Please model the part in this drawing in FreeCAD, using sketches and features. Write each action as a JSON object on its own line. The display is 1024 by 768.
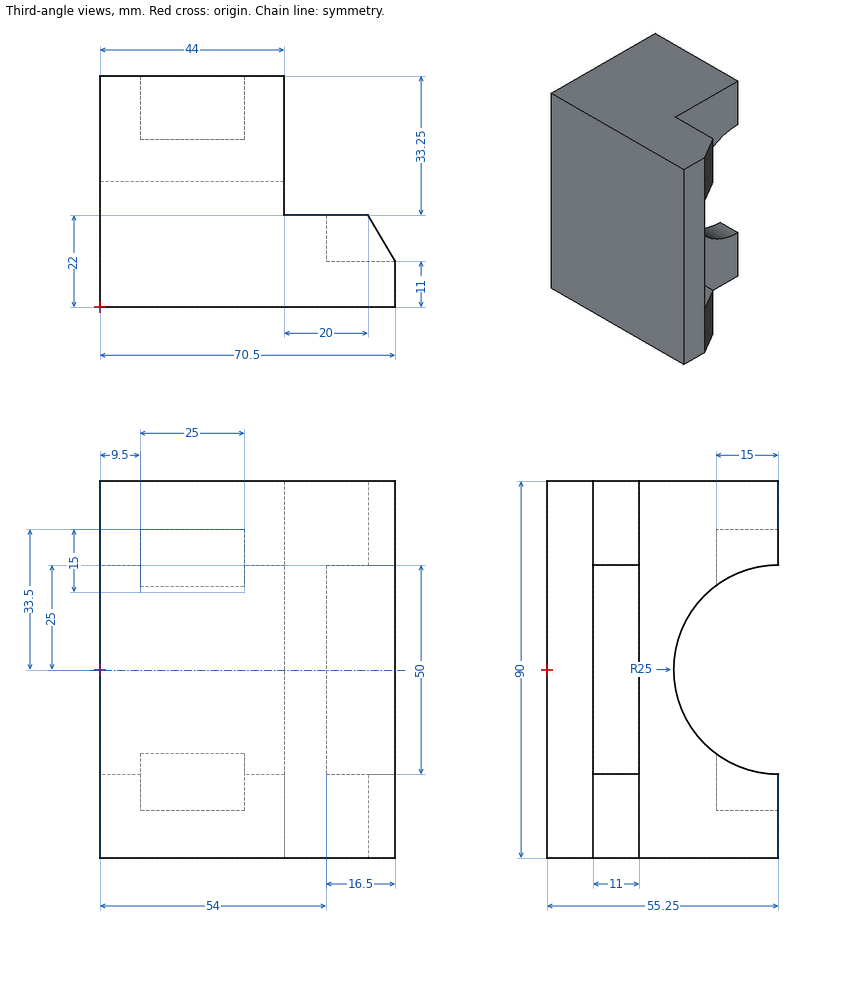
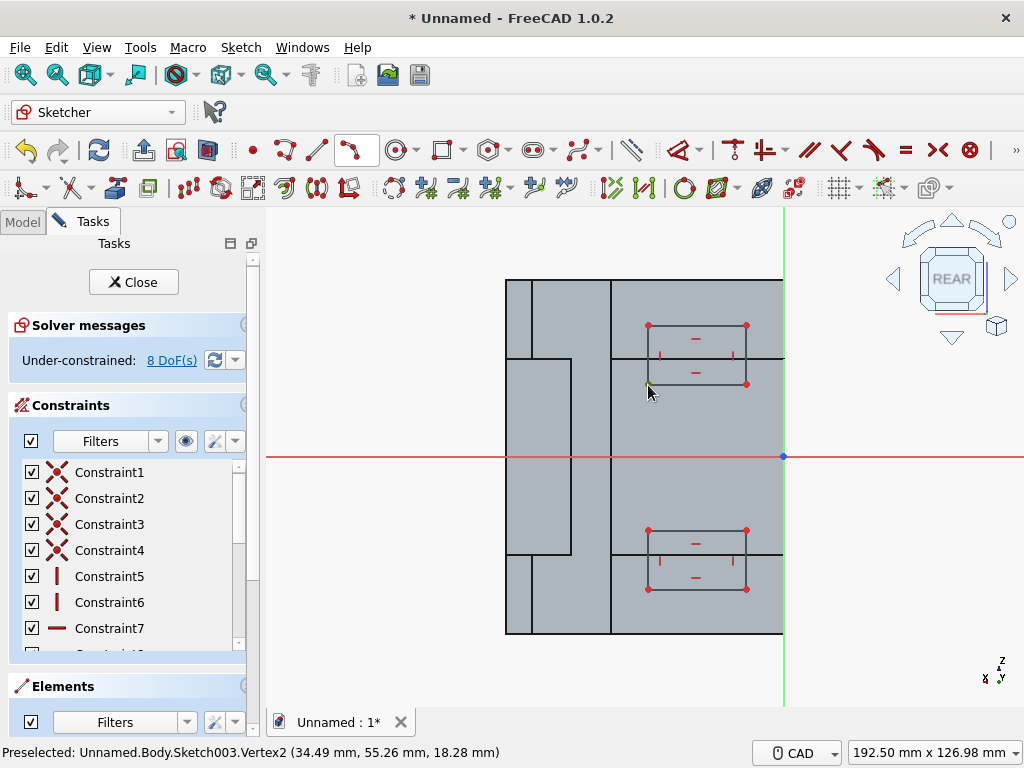
{"action": "left_click", "coordinate": [648, 531]}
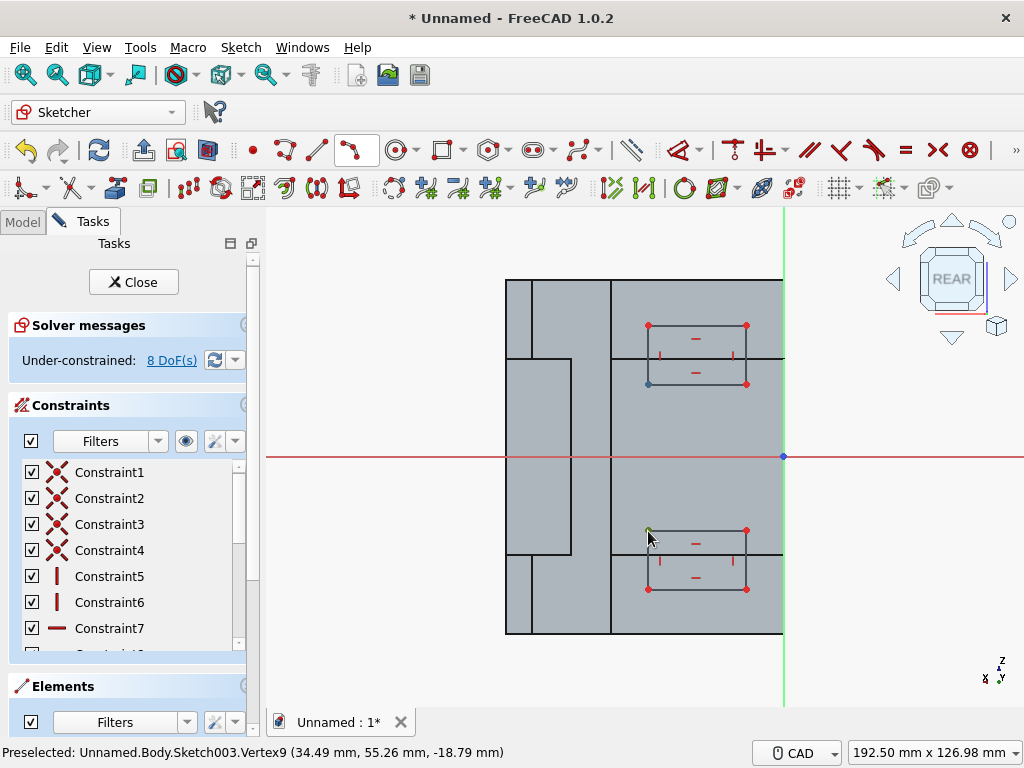
{"action": "left_click", "coordinate": [334, 457]}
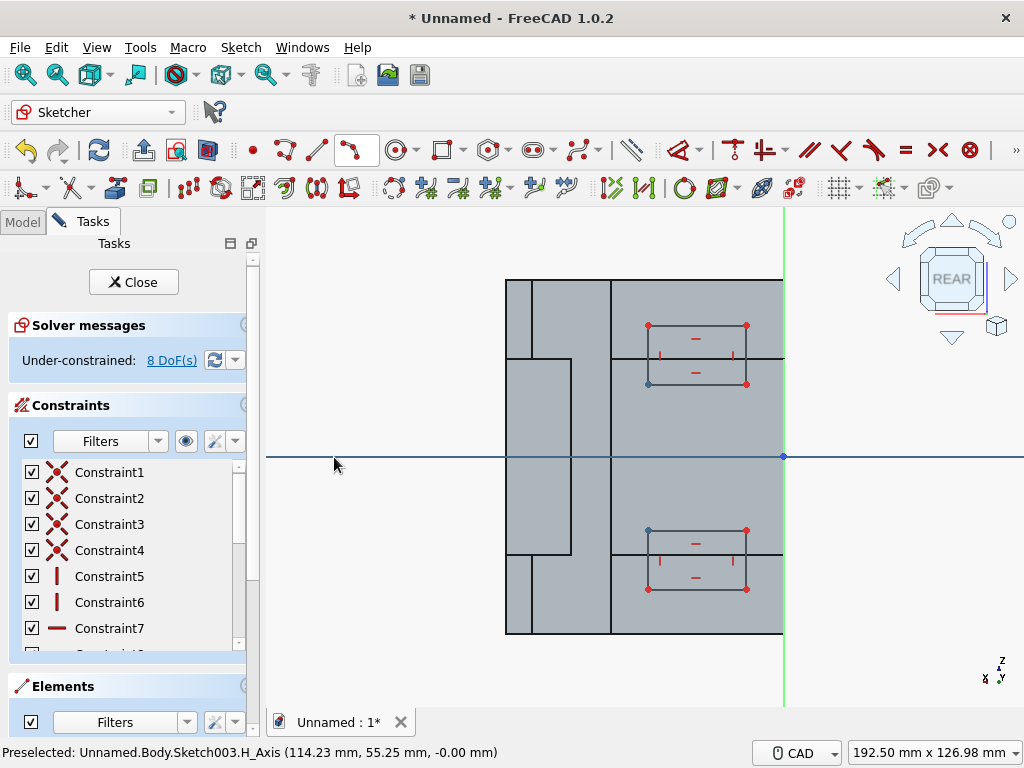
{"action": "left_click", "coordinate": [938, 150]}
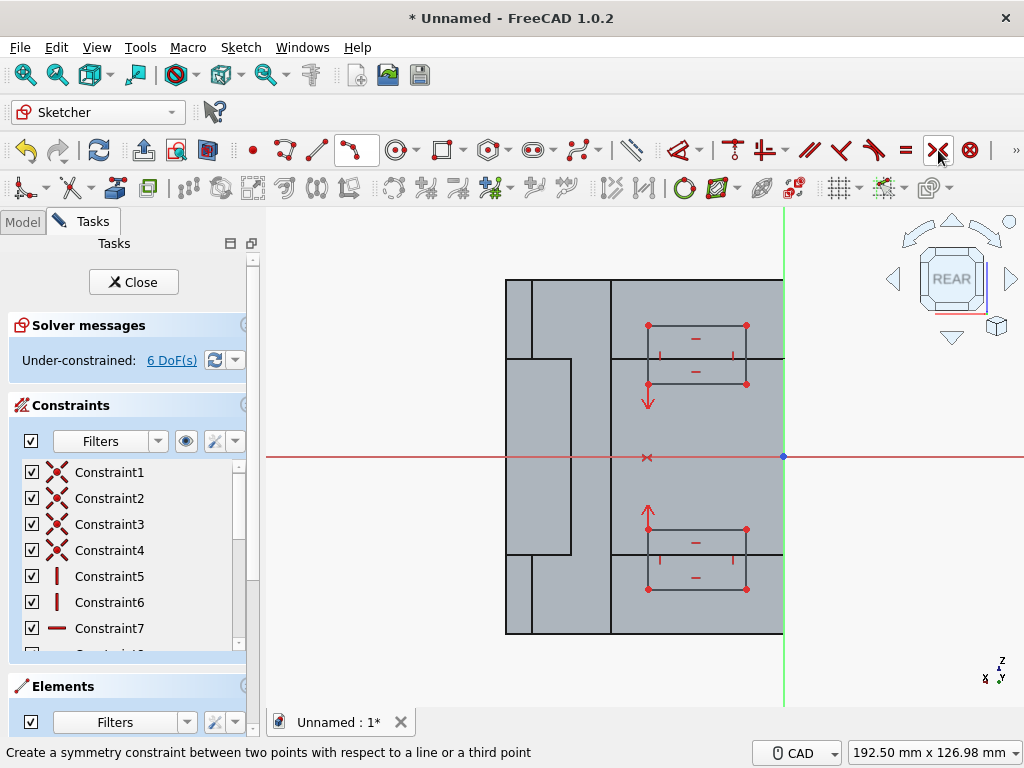
{"action": "left_click", "coordinate": [746, 326]}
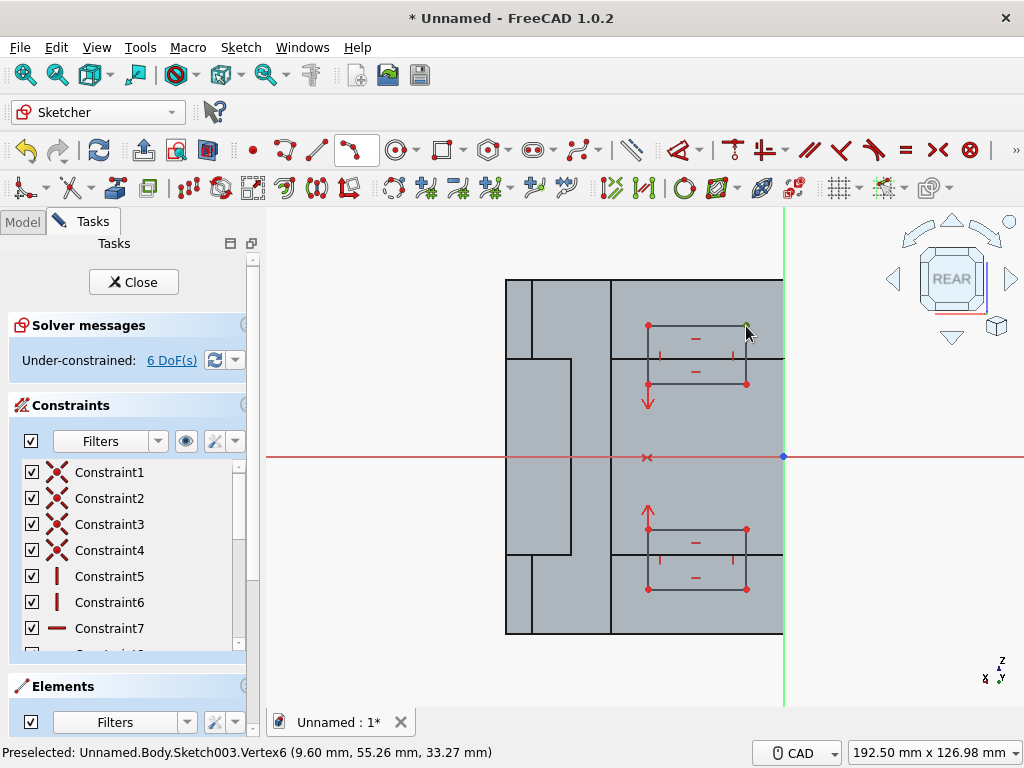
{"action": "left_click", "coordinate": [746, 590]}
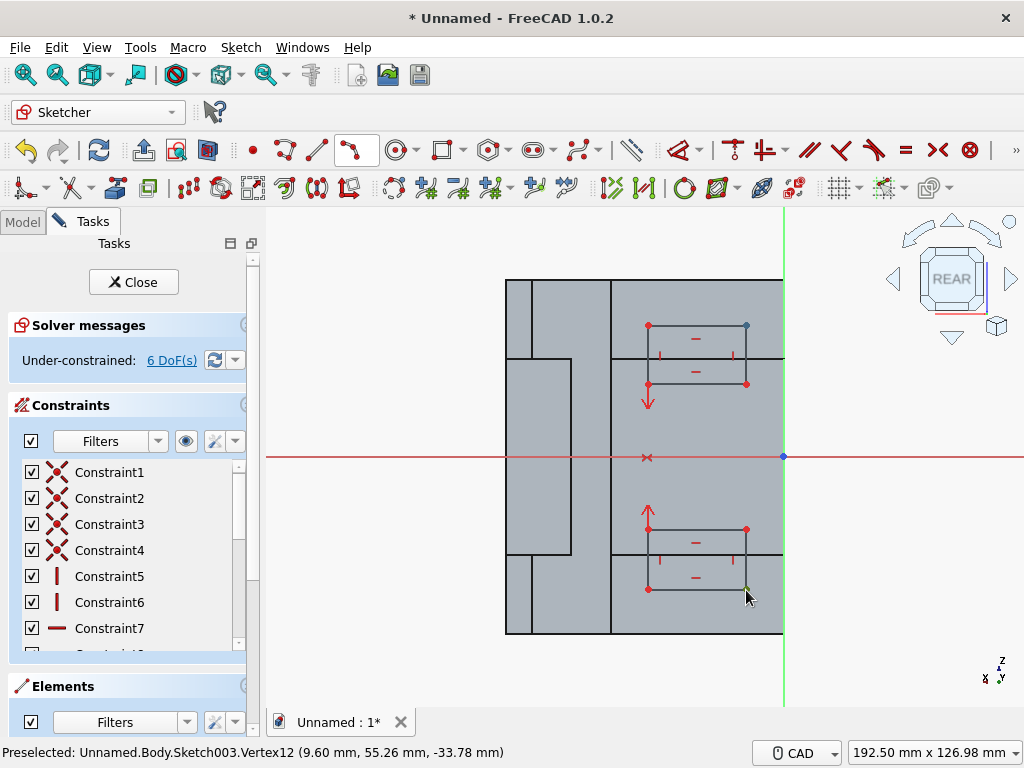
{"action": "left_click", "coordinate": [334, 457]}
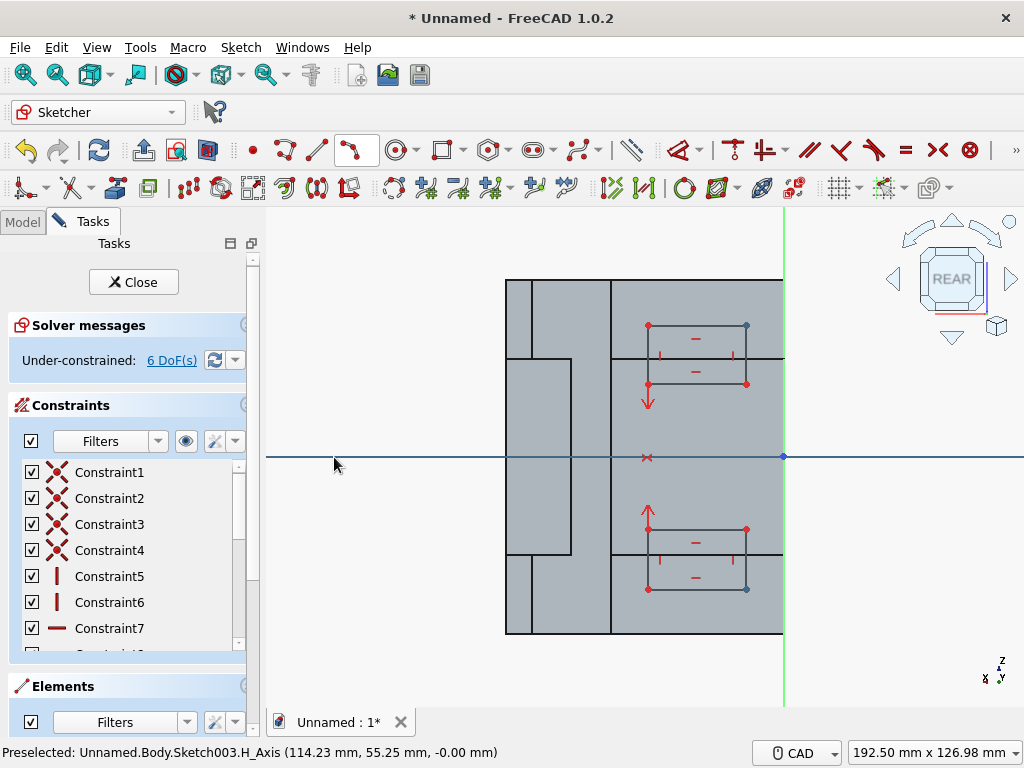
{"action": "left_click", "coordinate": [938, 150]}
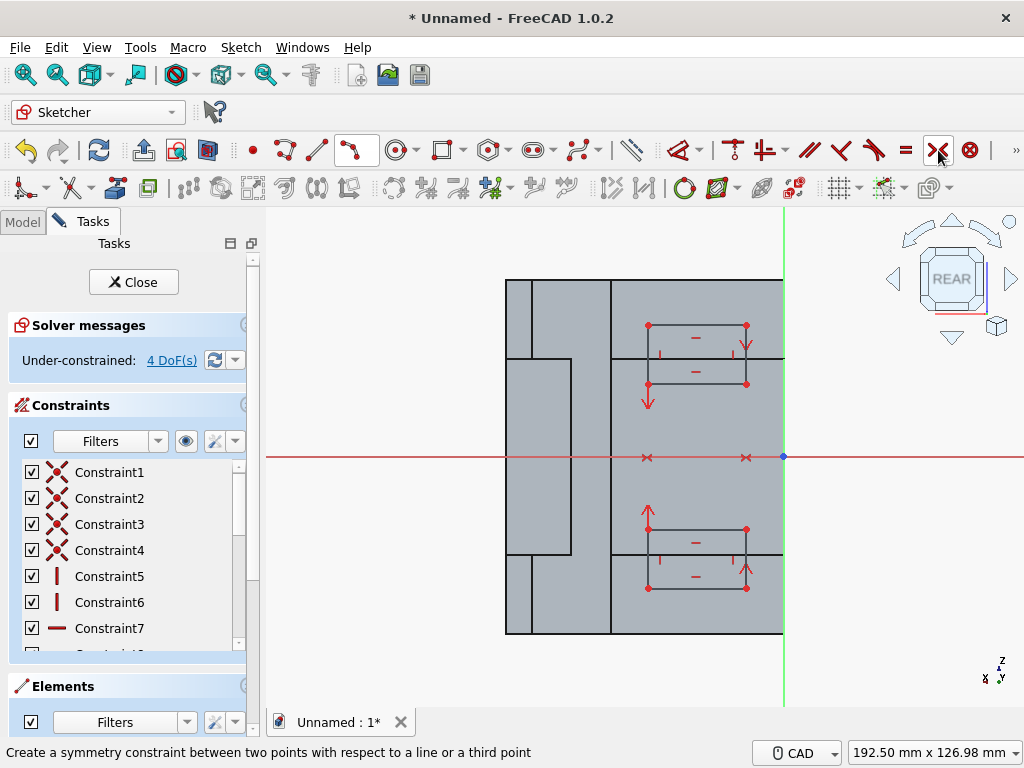
{"action": "left_click", "coordinate": [678, 150]}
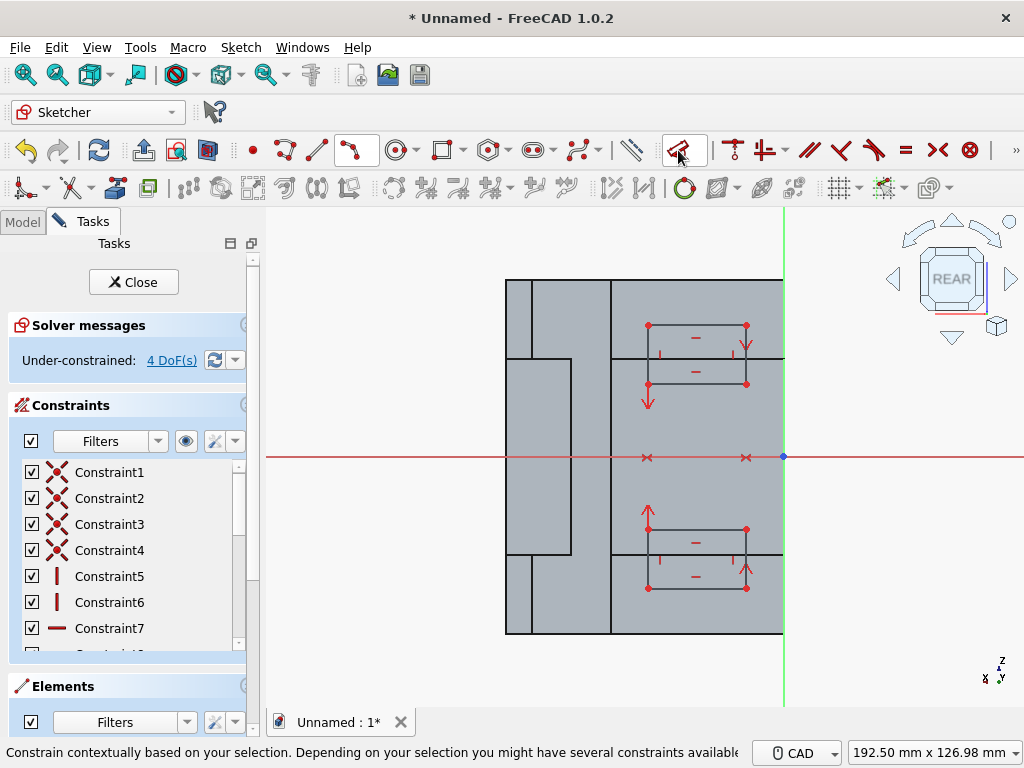
{"action": "left_click", "coordinate": [648, 343]}
{"action": "left_click", "coordinate": [614, 355]}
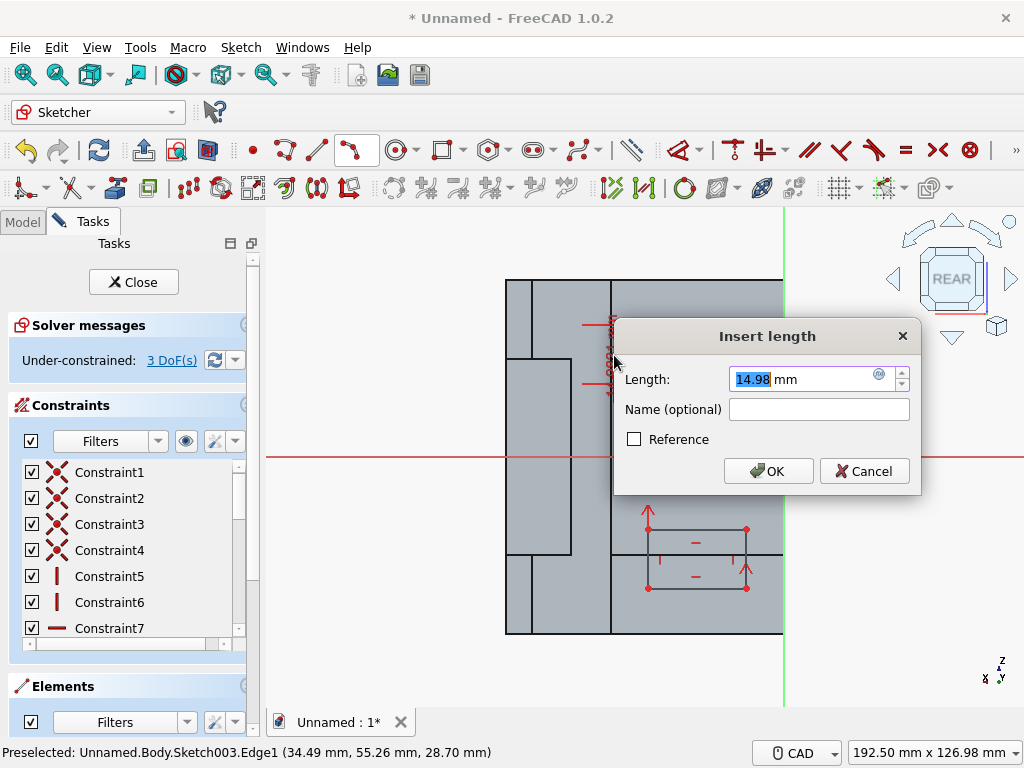
{"action": "type", "text": "15"}
{"action": "key", "text": "Return"}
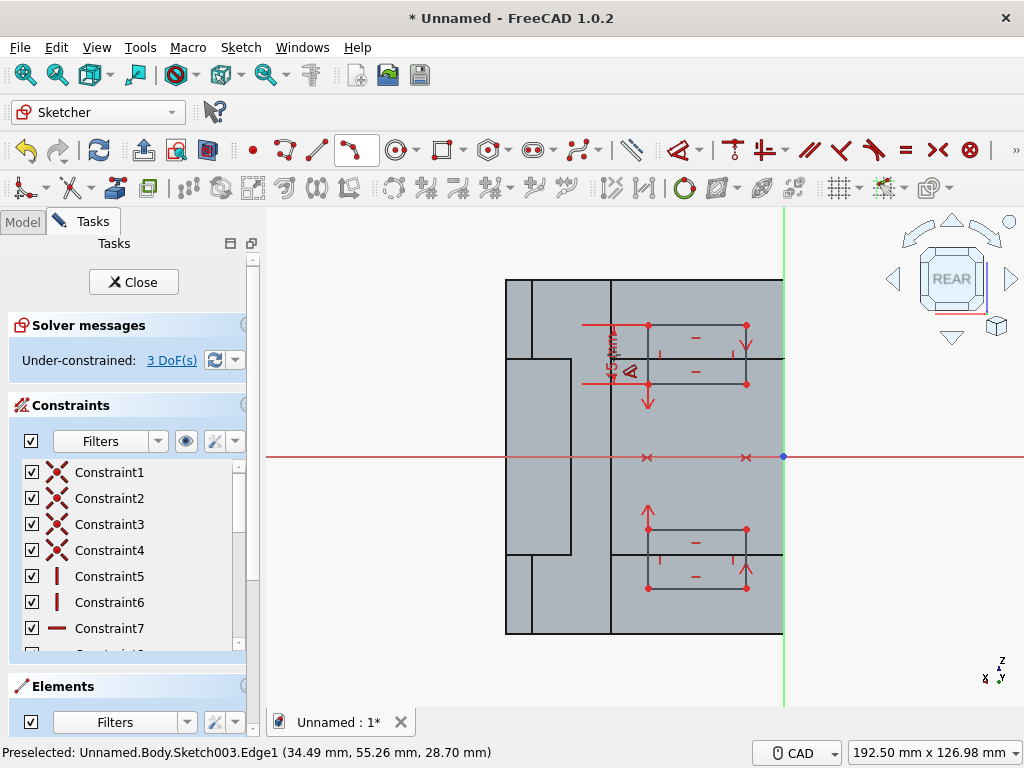
{"action": "left_click", "coordinate": [677, 384]}
{"action": "left_click", "coordinate": [697, 350]}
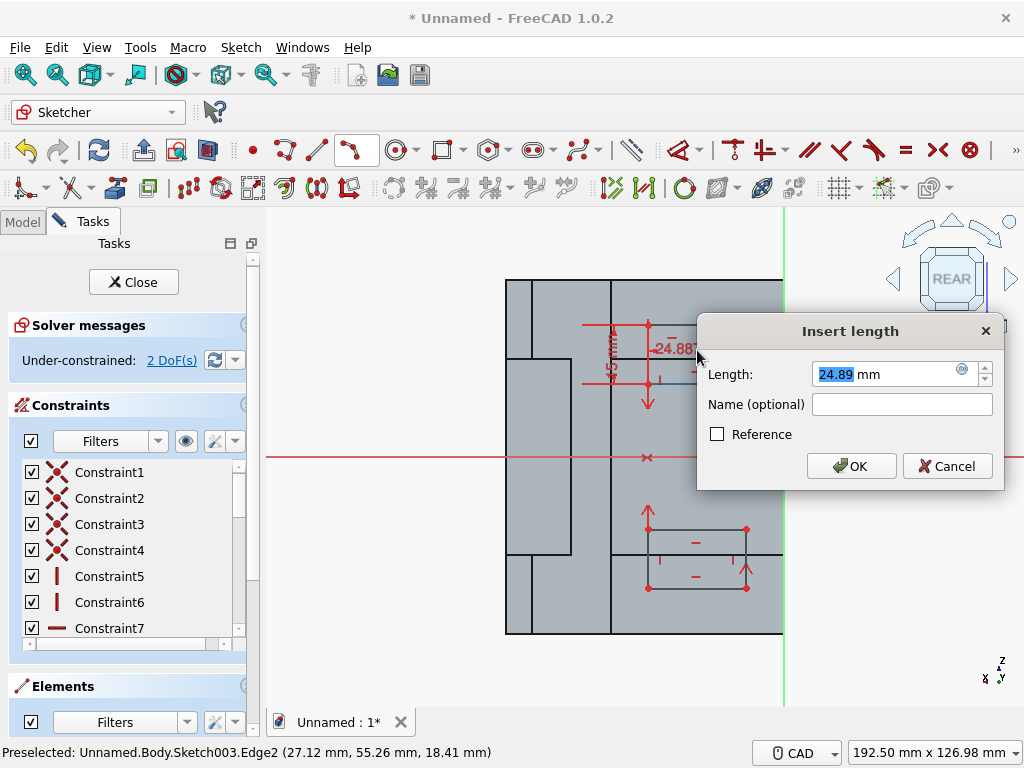
{"action": "type", "text": "25"}
{"action": "key", "text": "Return"}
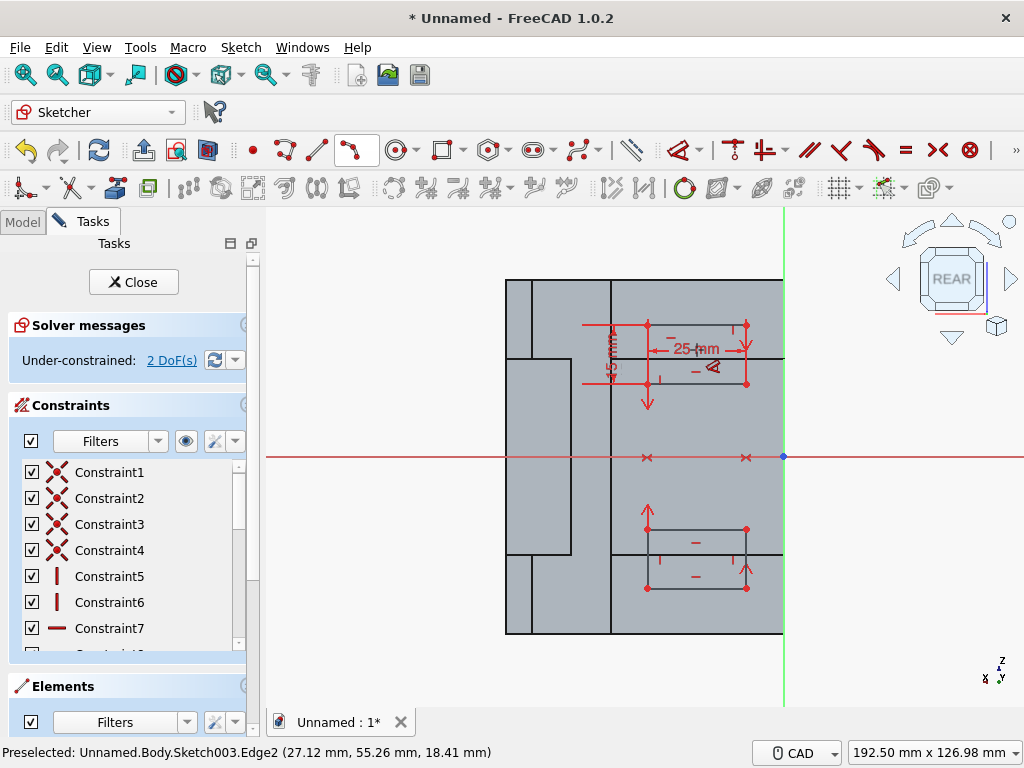
{"action": "left_click", "coordinate": [746, 384]}
{"action": "left_click", "coordinate": [765, 491]}